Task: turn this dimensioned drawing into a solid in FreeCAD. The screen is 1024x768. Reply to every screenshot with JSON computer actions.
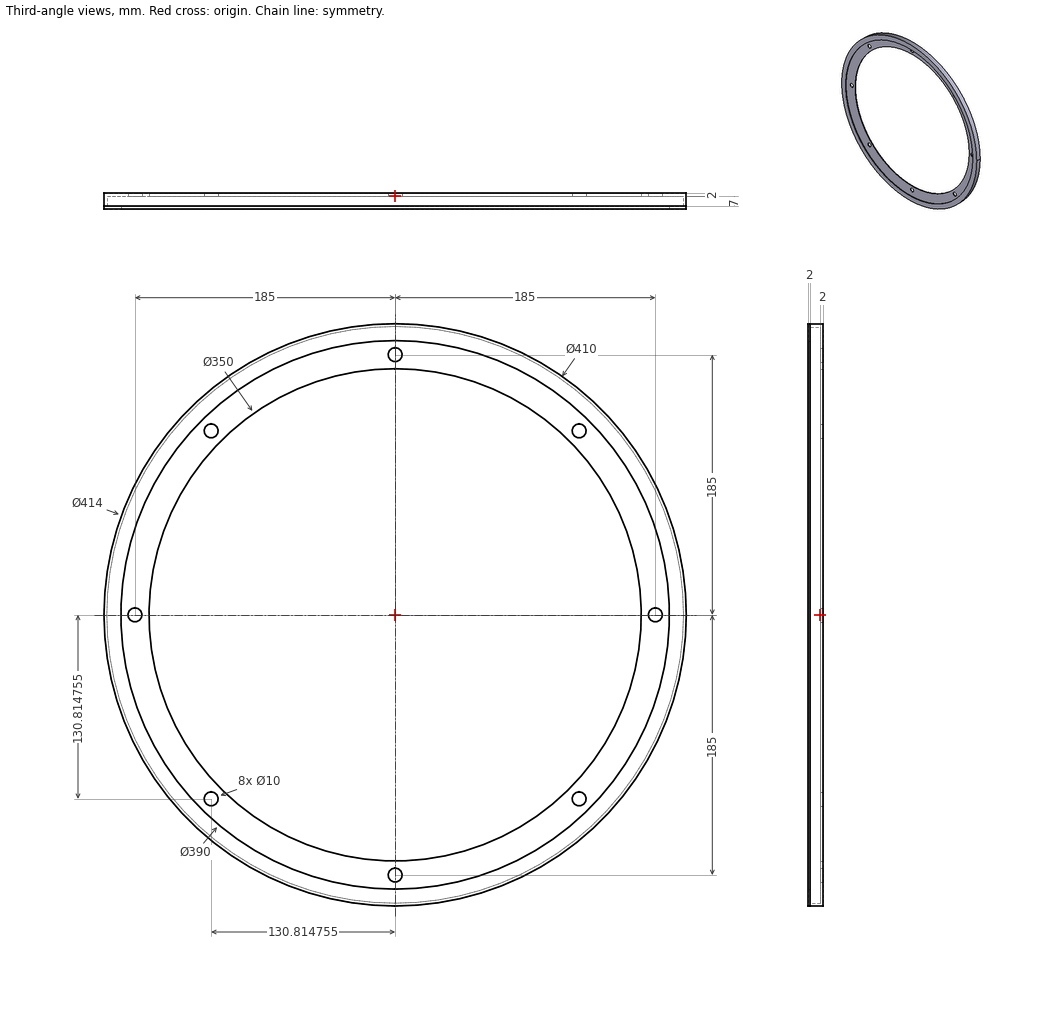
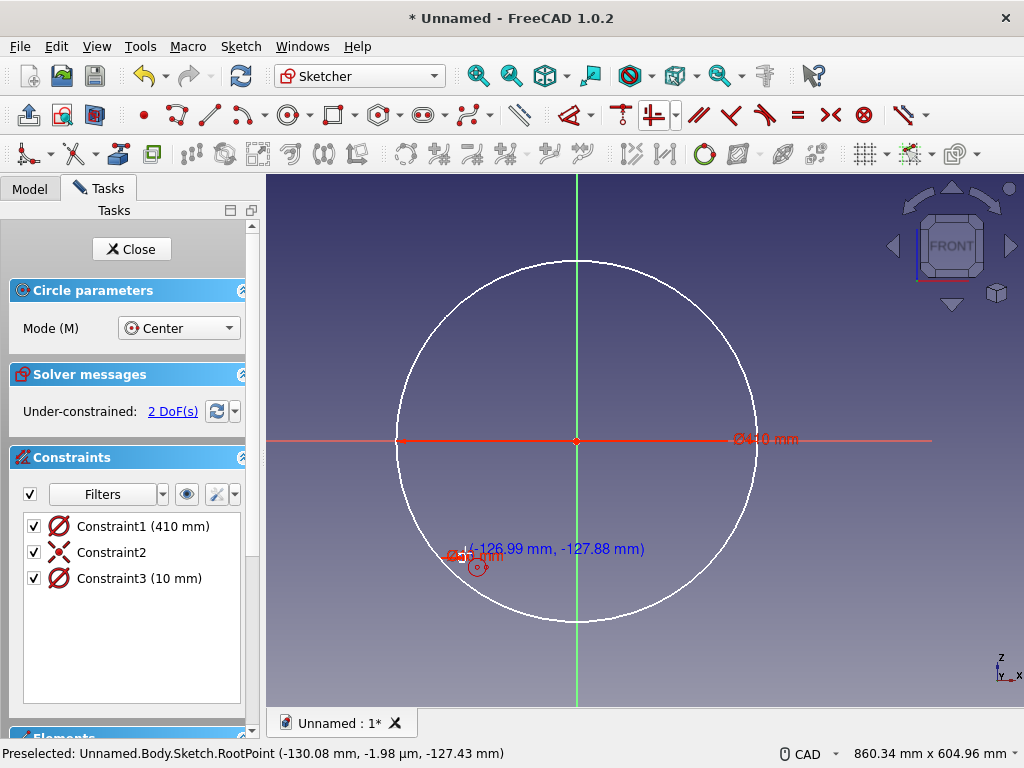
{"action": "scroll", "coordinate": [577, 604], "scroll_direction": "up", "scroll_amount": 9}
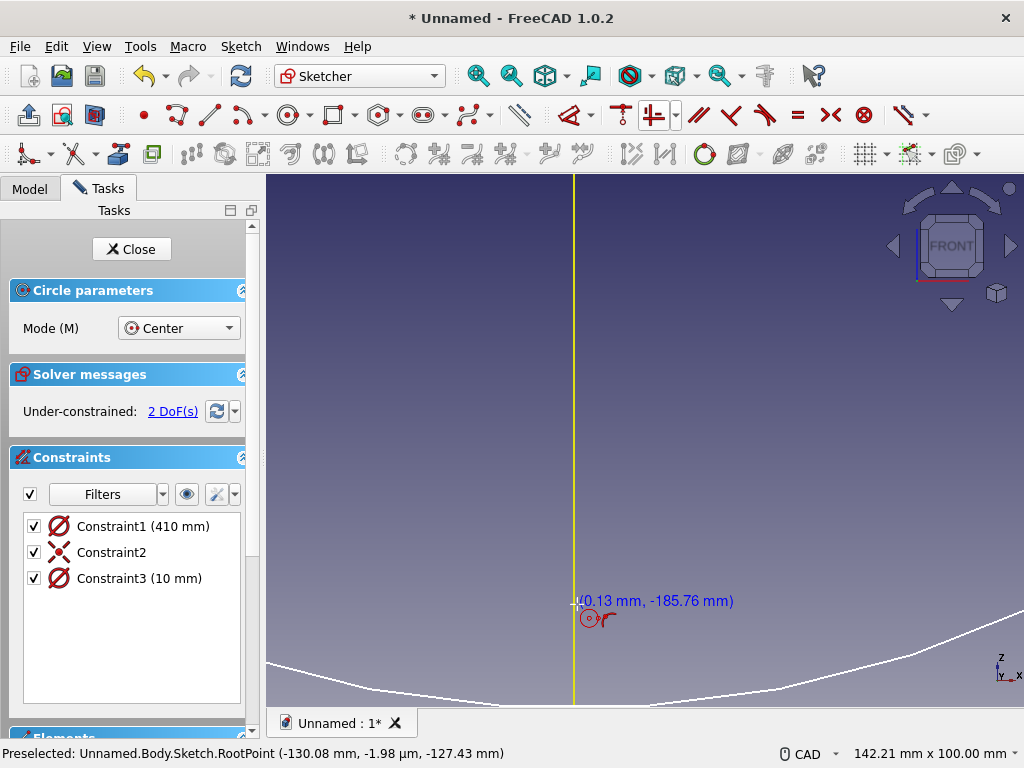
{"action": "scroll", "coordinate": [577, 604], "scroll_direction": "down", "scroll_amount": 9}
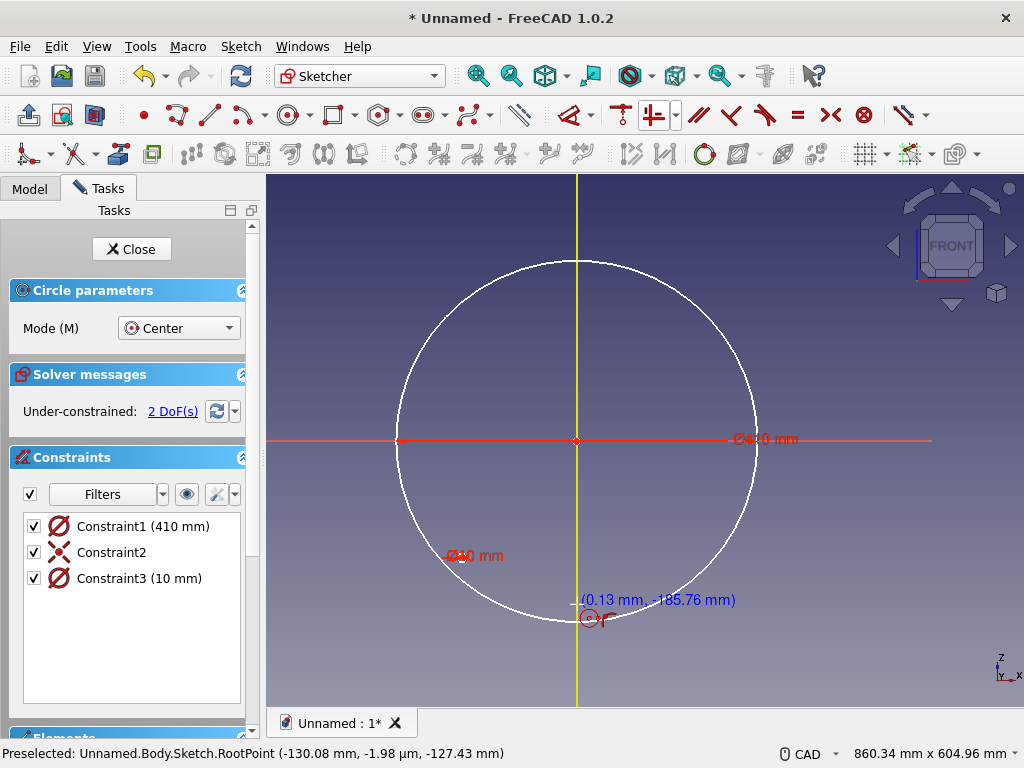
{"action": "left_click", "coordinate": [577, 604]}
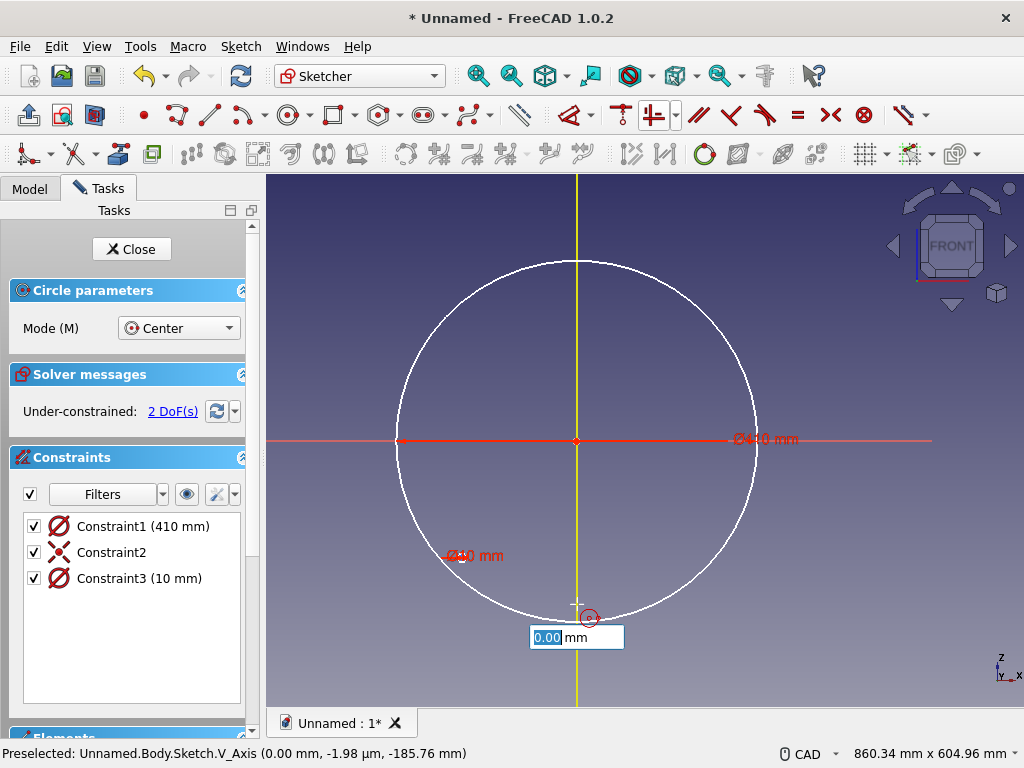
{"action": "scroll", "coordinate": [581, 603], "scroll_direction": "up", "scroll_amount": 7}
{"action": "mouse_move", "coordinate": [580, 600]}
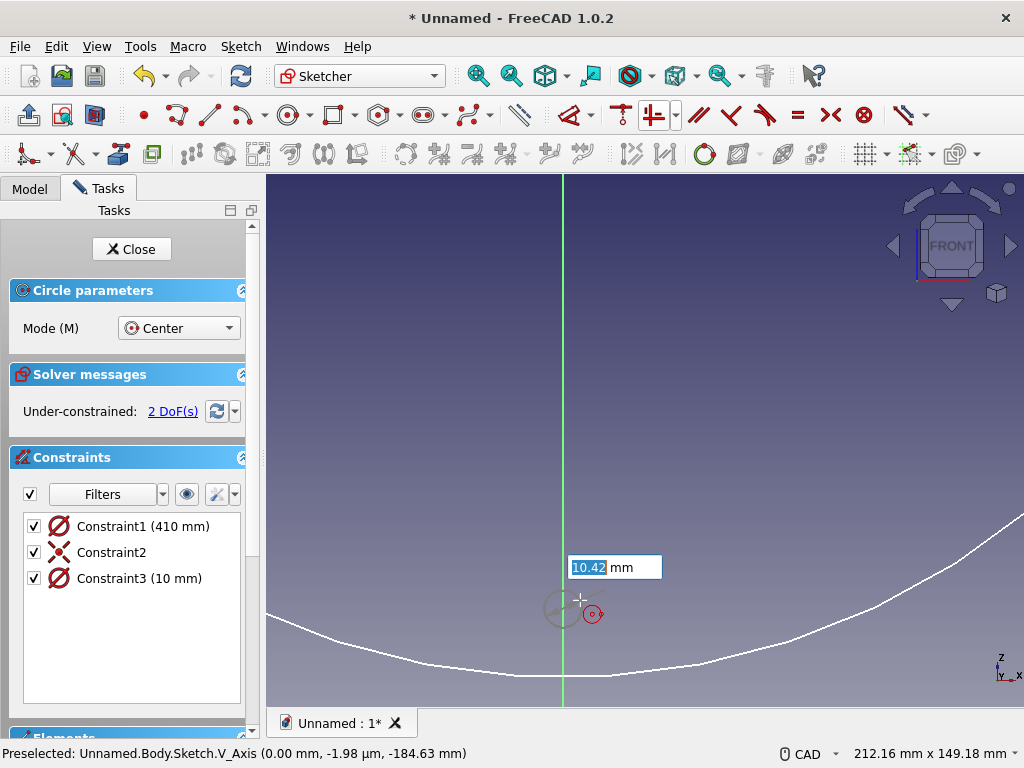
{"action": "type", "text": "10"}
{"action": "key", "text": "Return"}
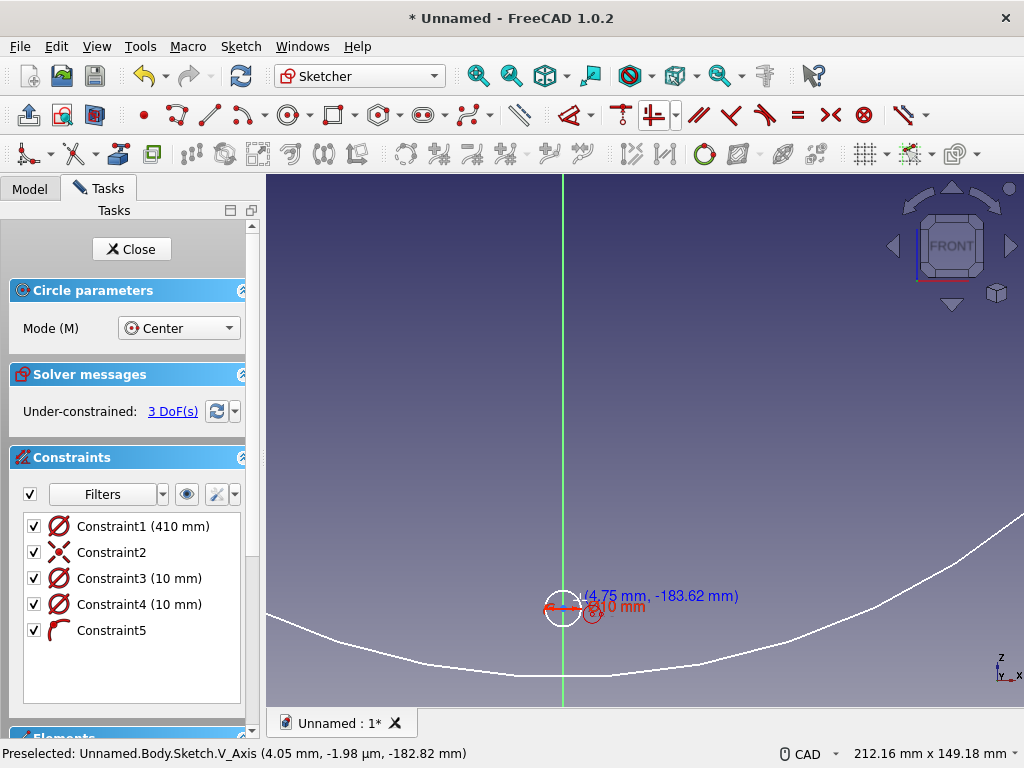
{"action": "scroll", "coordinate": [581, 603], "scroll_direction": "down", "scroll_amount": 7}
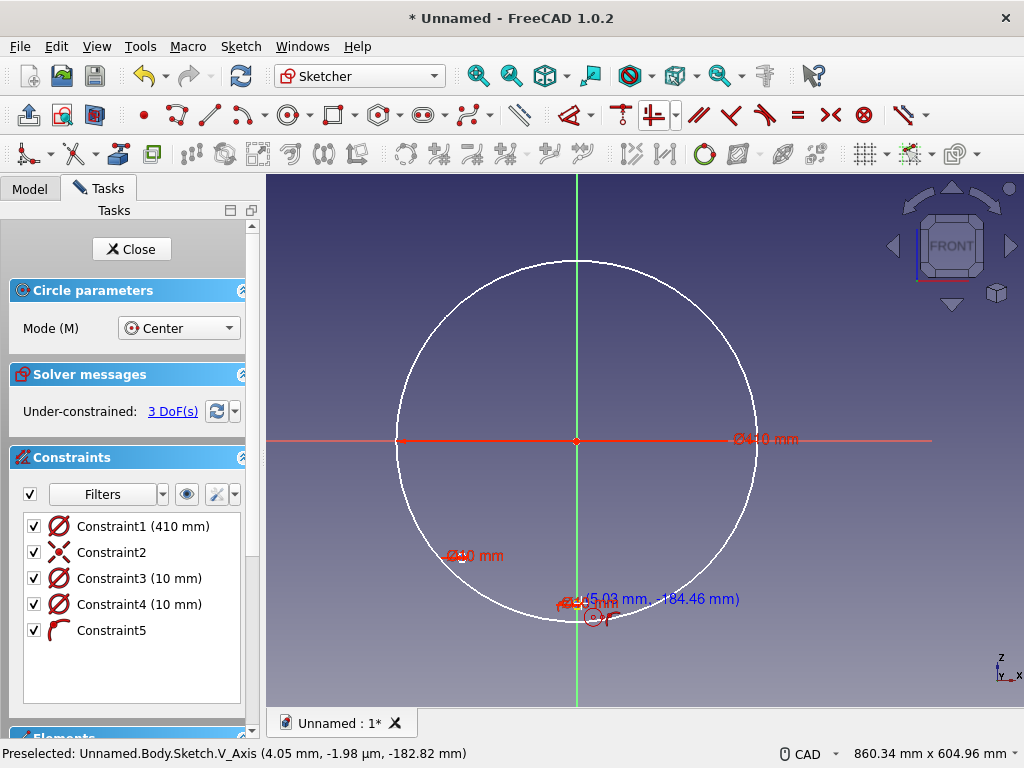
{"action": "scroll", "coordinate": [414, 441], "scroll_direction": "up", "scroll_amount": 9}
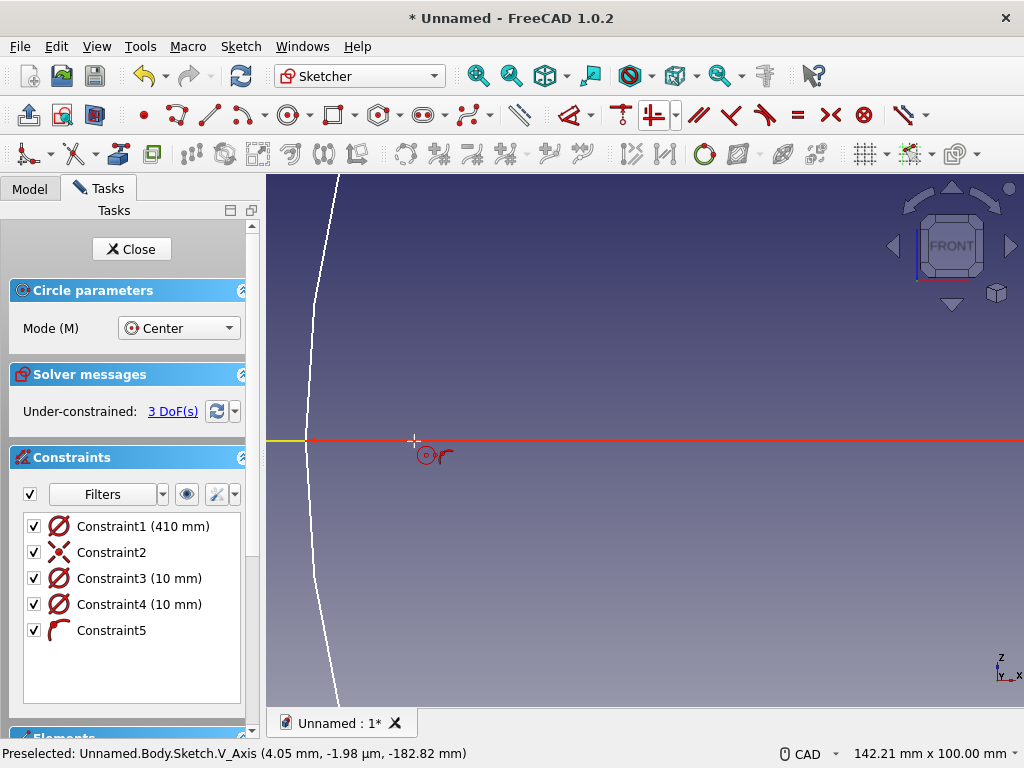
{"action": "scroll", "coordinate": [414, 440], "scroll_direction": "down", "scroll_amount": 9}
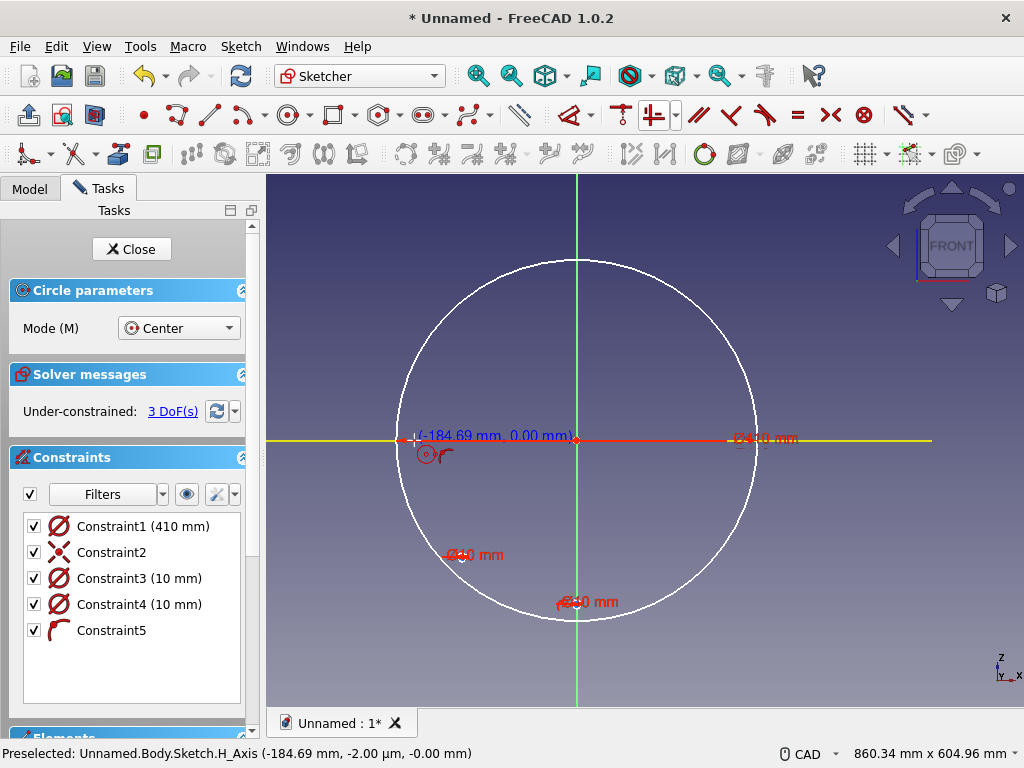
{"action": "left_click", "coordinate": [414, 441]}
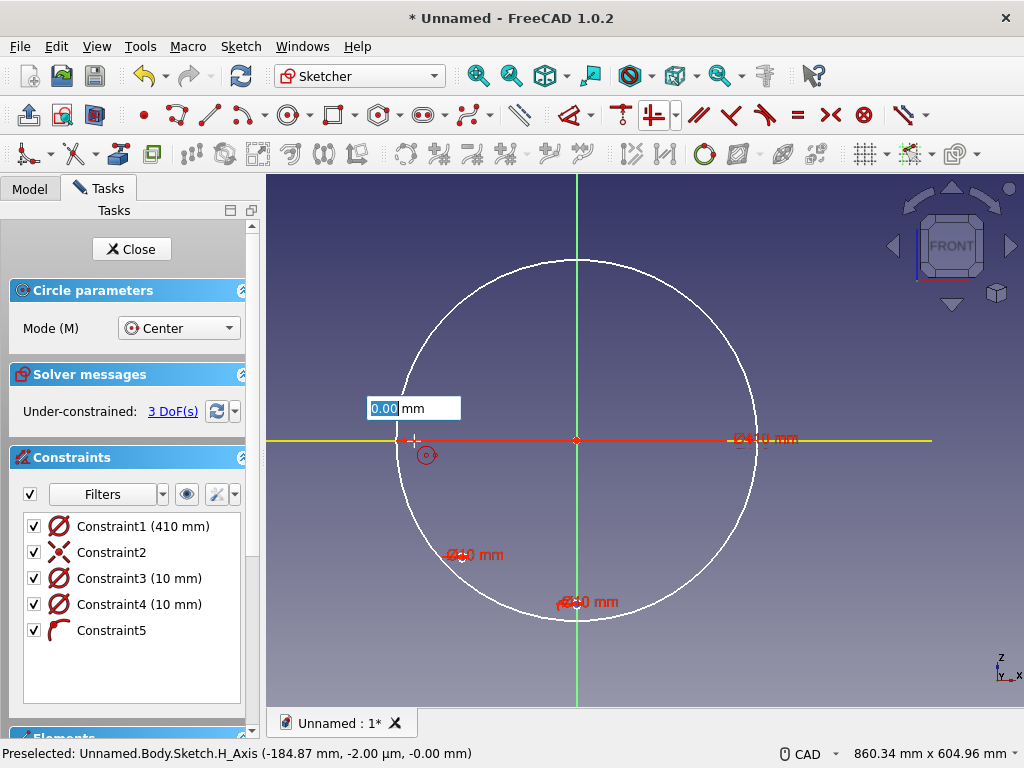
{"action": "scroll", "coordinate": [412, 445], "scroll_direction": "up", "scroll_amount": 7}
{"action": "mouse_move", "coordinate": [413, 442]}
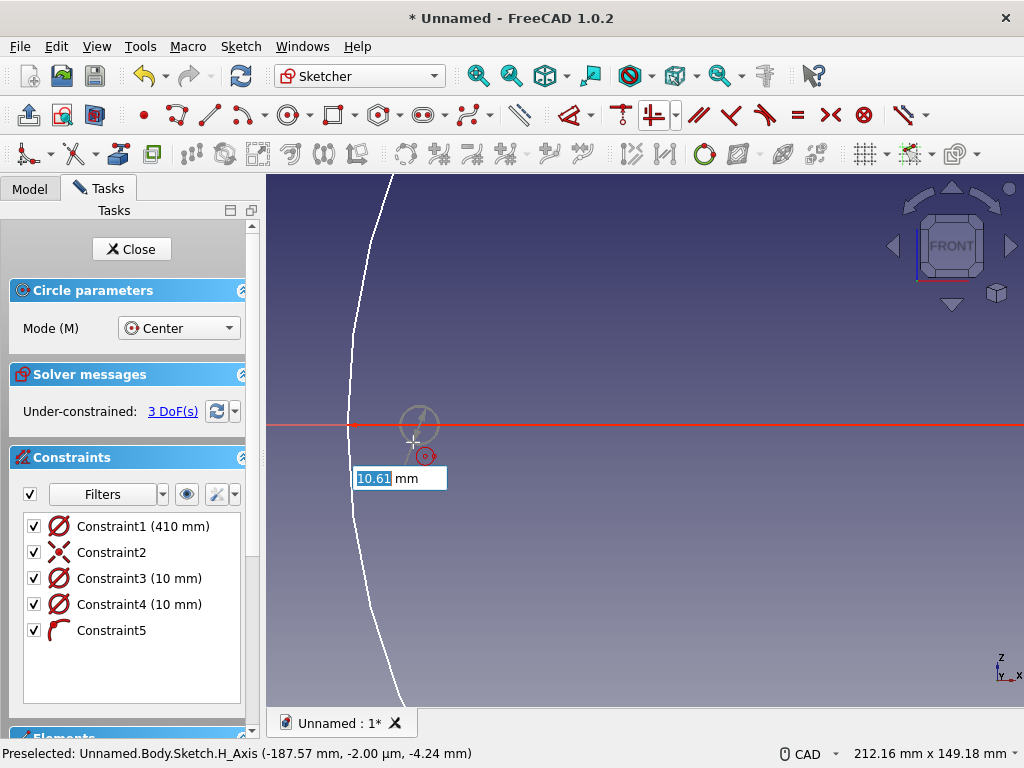
{"action": "type", "text": "10"}
{"action": "key", "text": "Return"}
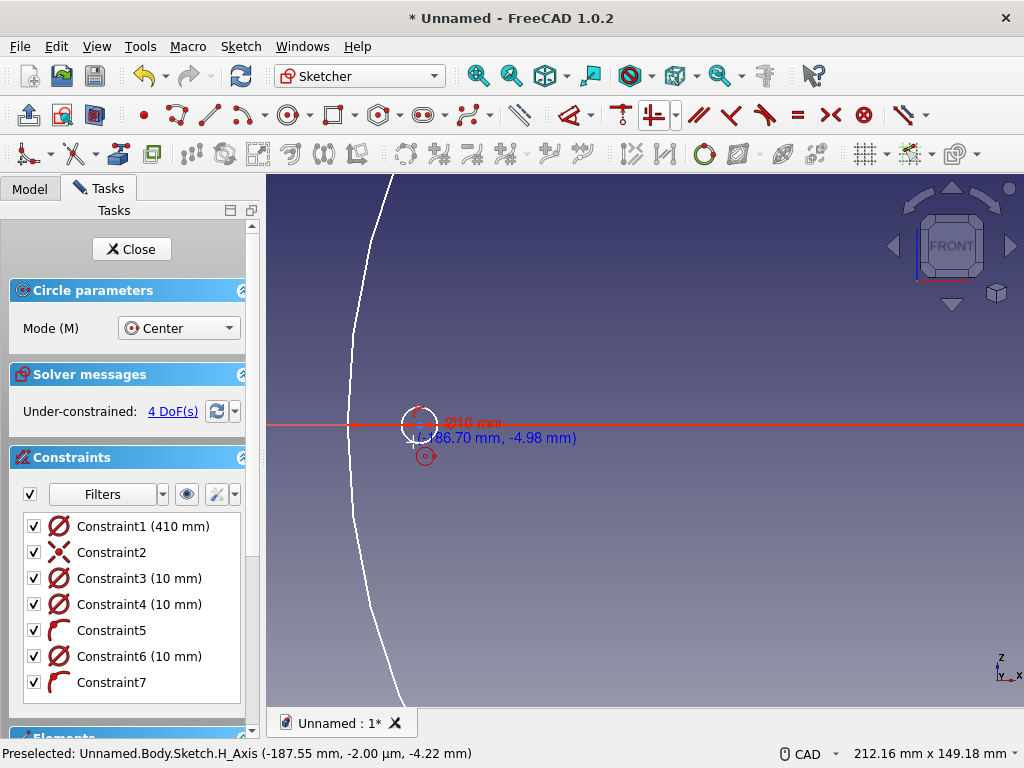
{"action": "scroll", "coordinate": [412, 446], "scroll_direction": "down", "scroll_amount": 7}